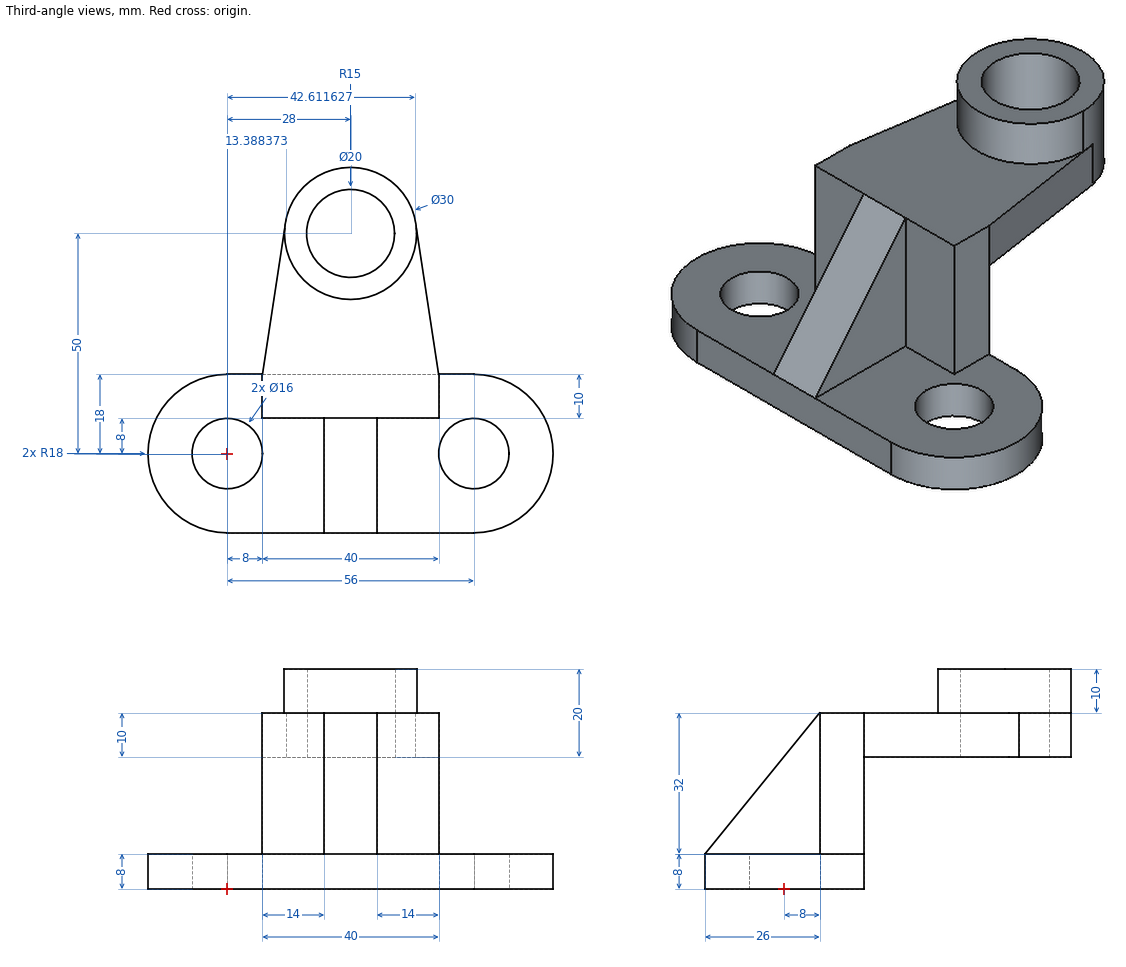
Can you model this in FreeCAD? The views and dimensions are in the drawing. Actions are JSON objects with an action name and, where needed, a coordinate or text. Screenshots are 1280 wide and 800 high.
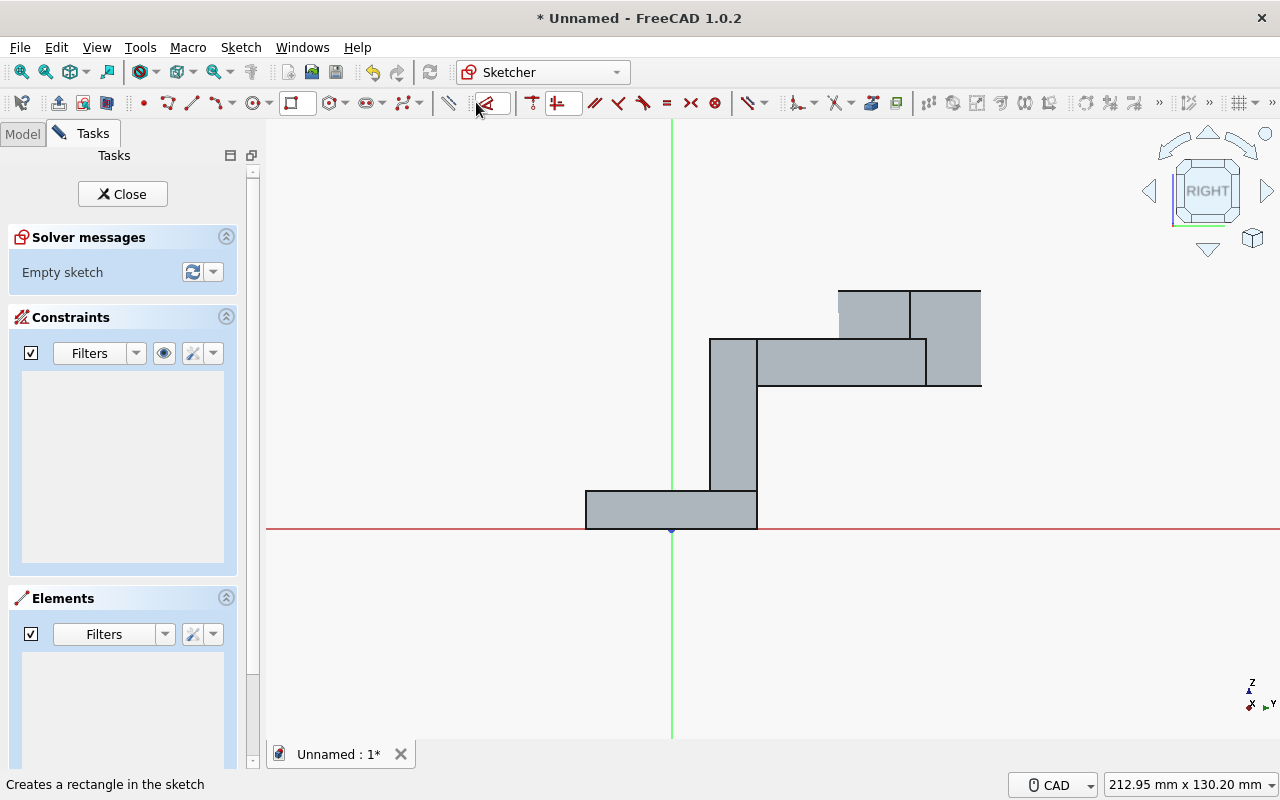
{"action": "key", "text": "q s"}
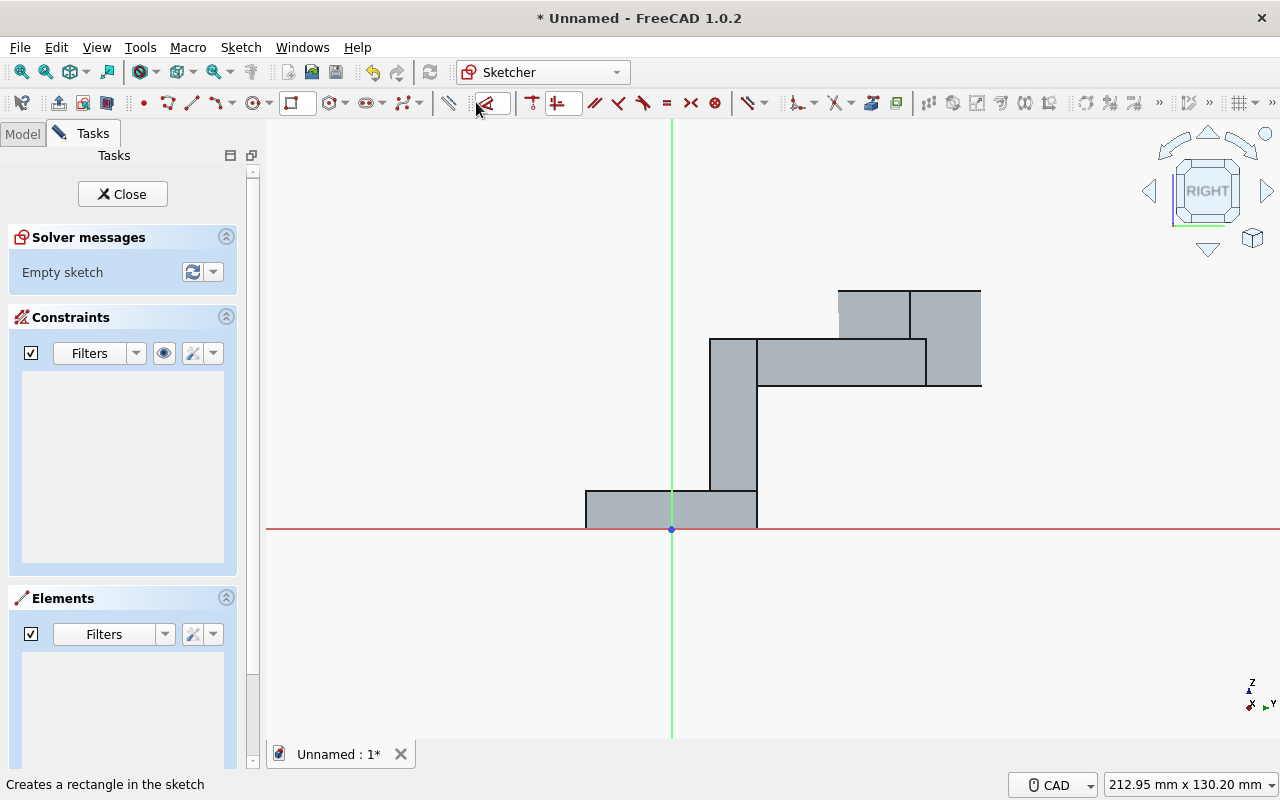
{"action": "scroll", "coordinate": [602, 438], "scroll_direction": "up", "scroll_amount": 4}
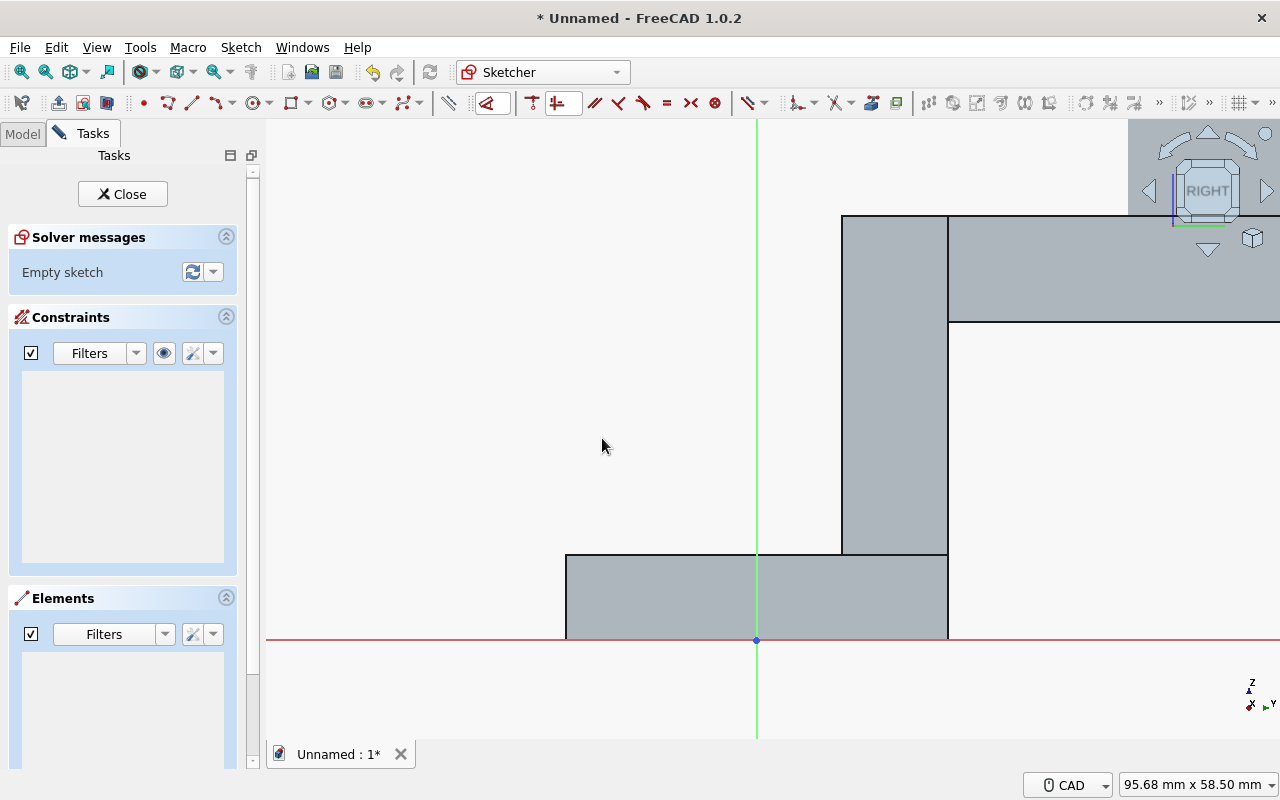
{"action": "left_click", "coordinate": [168, 104]}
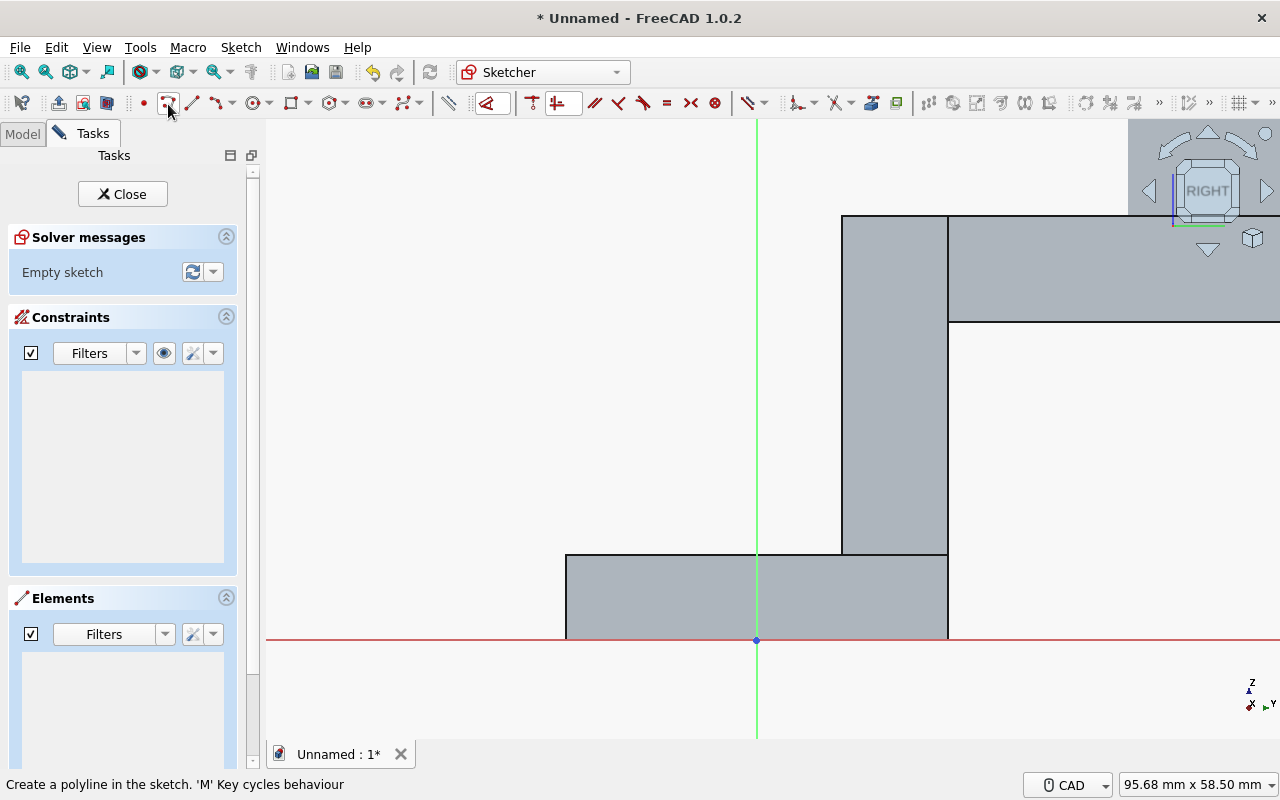
{"action": "left_click", "coordinate": [842, 555]}
{"action": "left_click", "coordinate": [842, 216]}
{"action": "left_click", "coordinate": [566, 555]}
{"action": "left_click", "coordinate": [842, 556]}
{"action": "key", "text": "Escape"}
{"action": "key", "text": "Escape"}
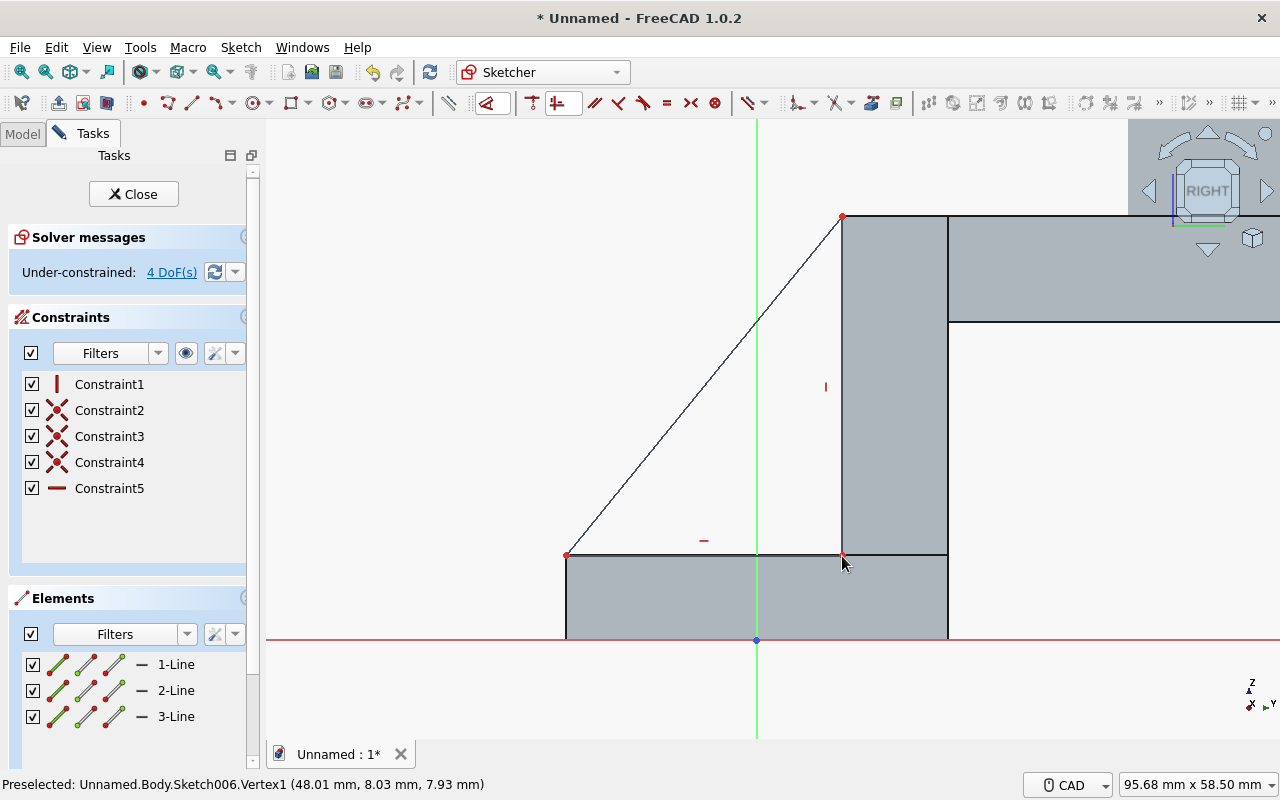
{"action": "left_click", "coordinate": [842, 454]}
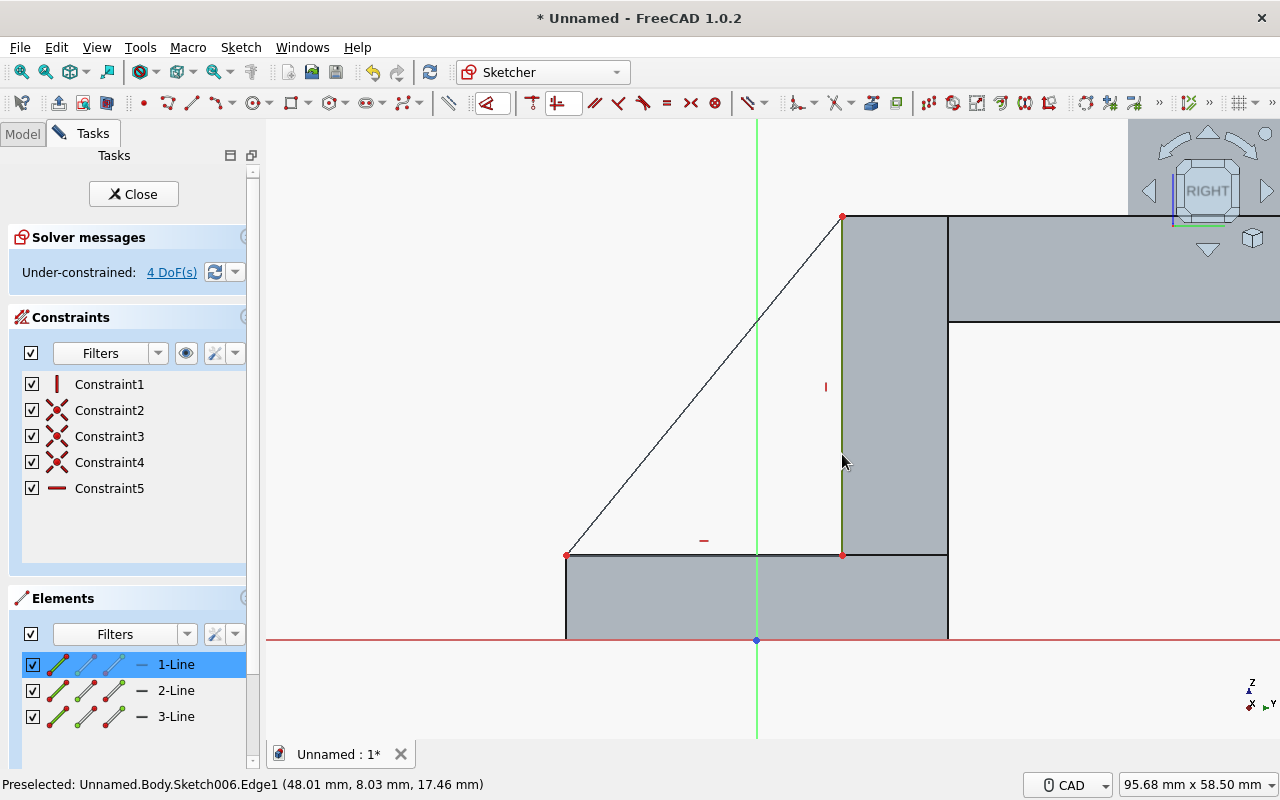
{"action": "left_click", "coordinate": [504, 104]}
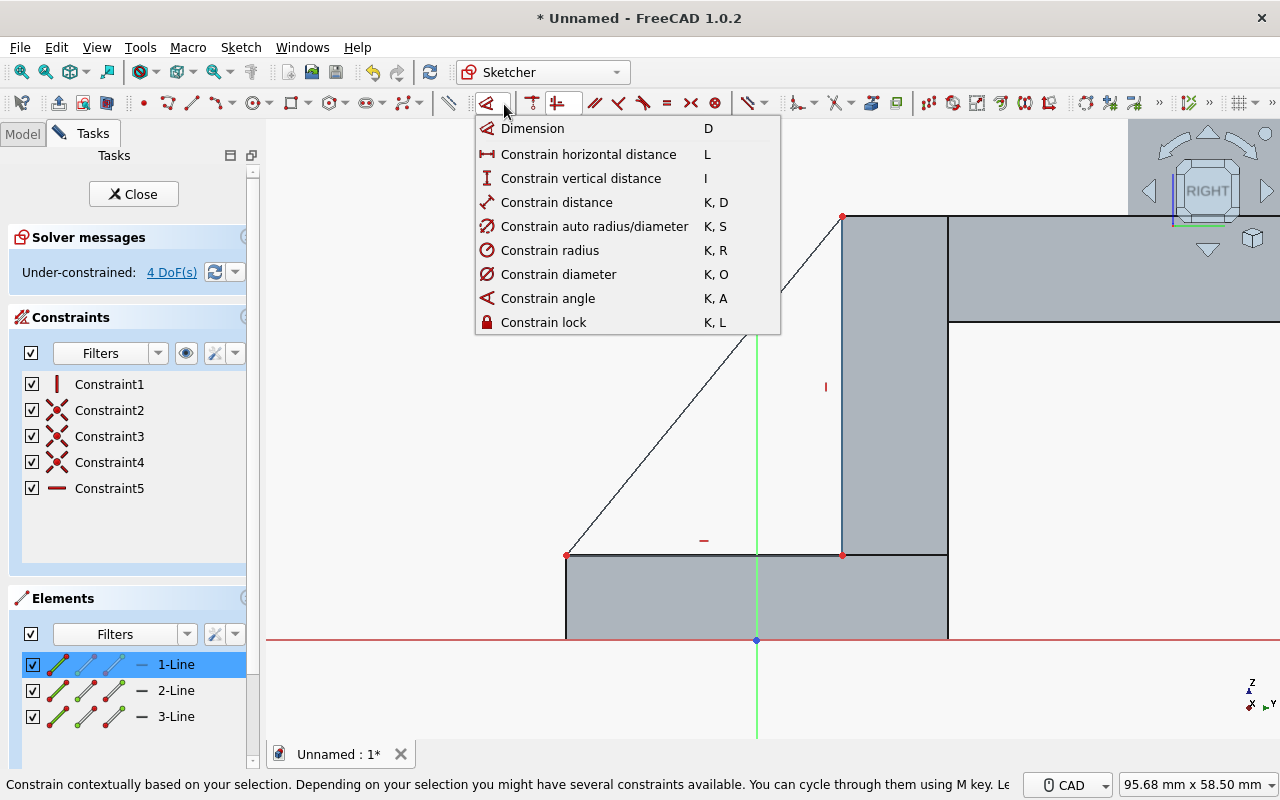
{"action": "left_click", "coordinate": [628, 178]}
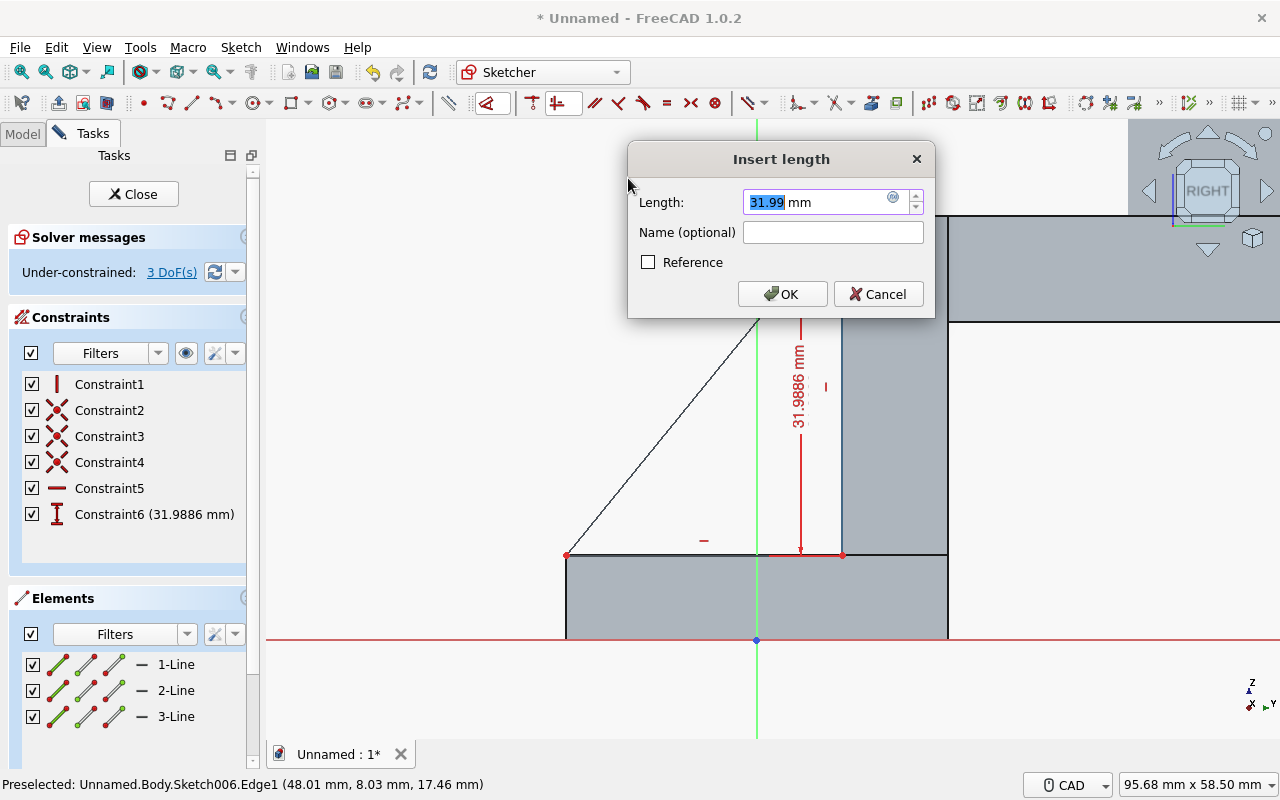
{"action": "type", "text": "32"}
{"action": "key", "text": "Return"}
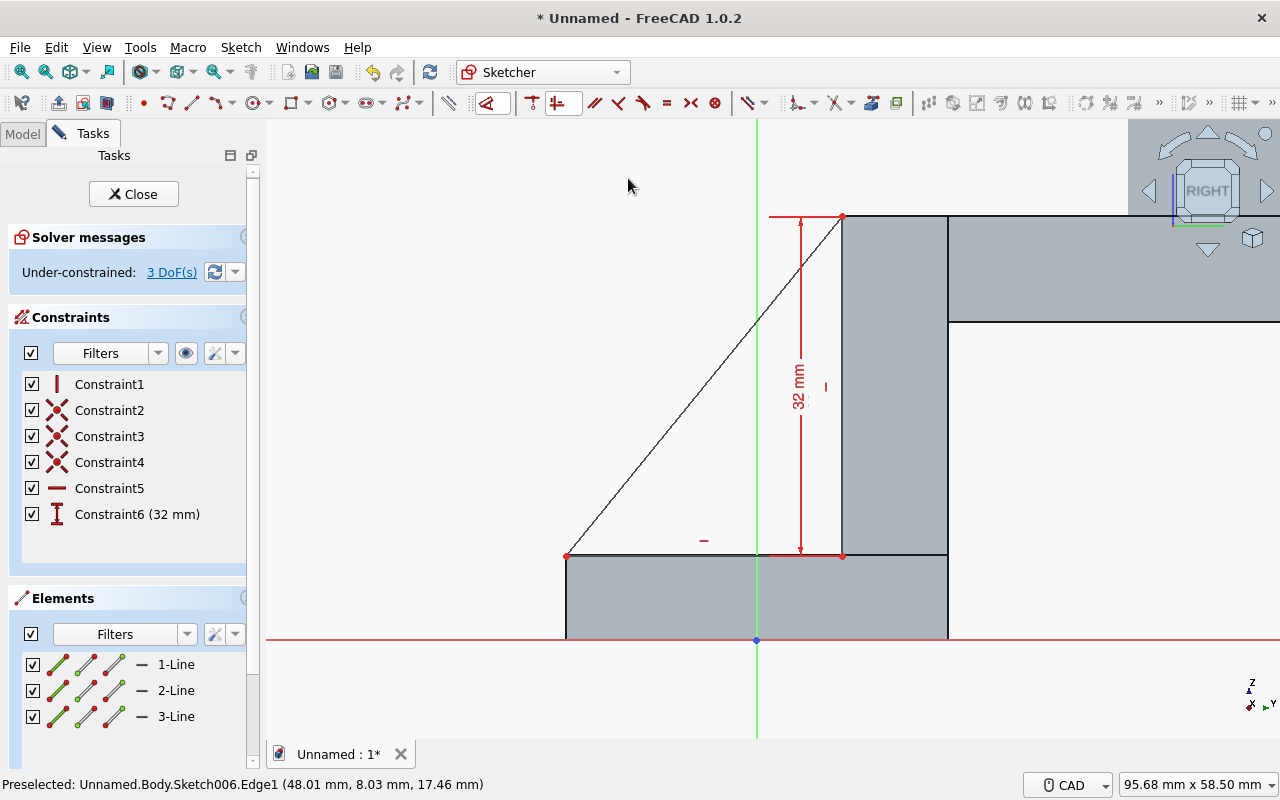
{"action": "left_click", "coordinate": [649, 556]}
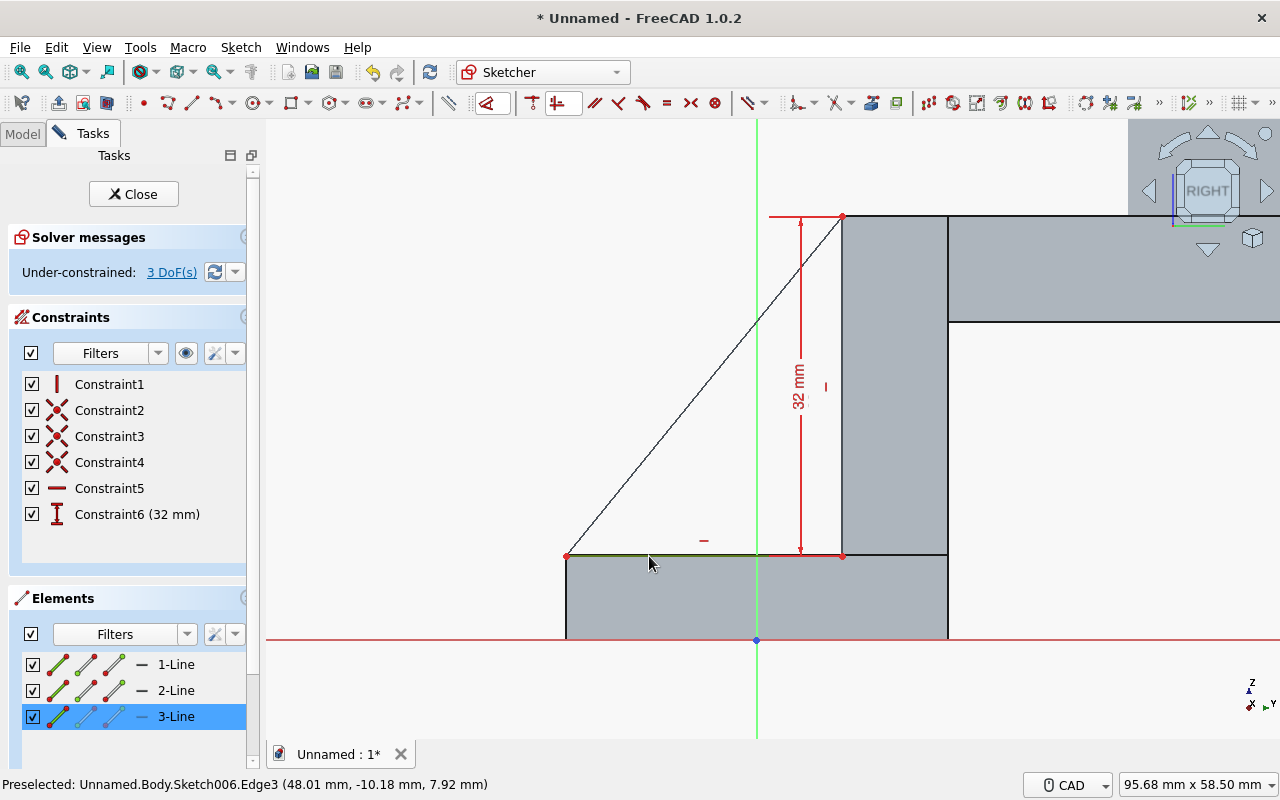
{"action": "left_click", "coordinate": [504, 104]}